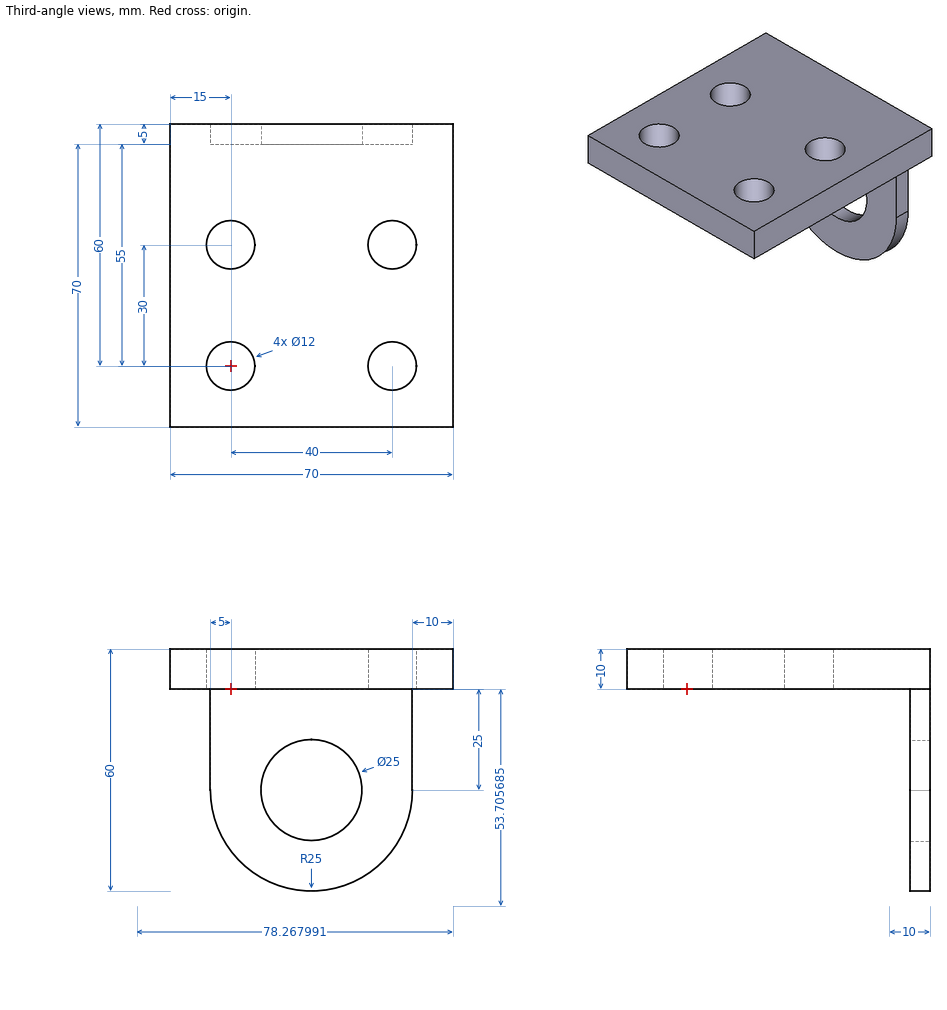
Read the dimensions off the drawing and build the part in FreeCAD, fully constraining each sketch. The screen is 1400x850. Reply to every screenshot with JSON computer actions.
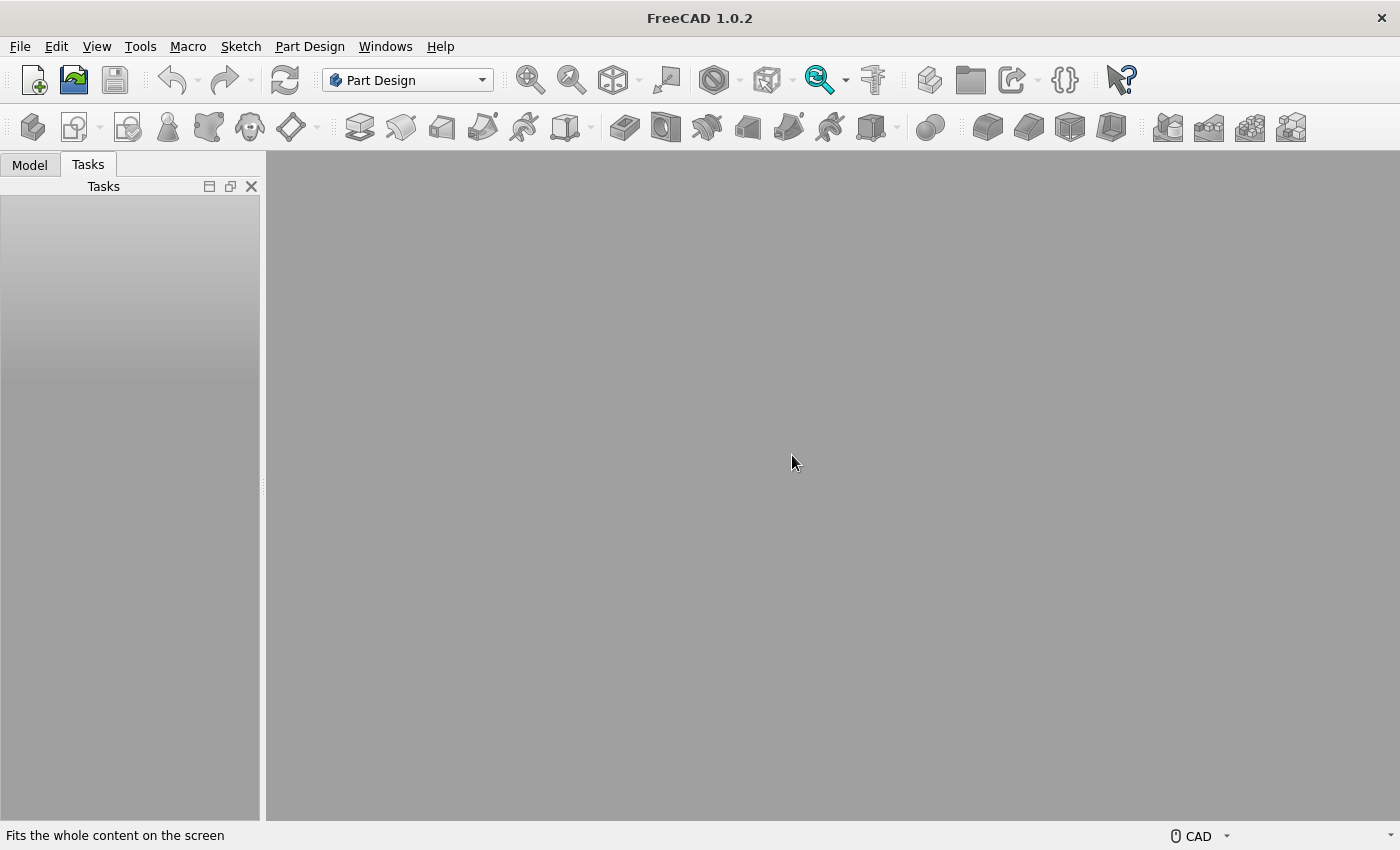
{"action": "key", "text": "ctrl+n"}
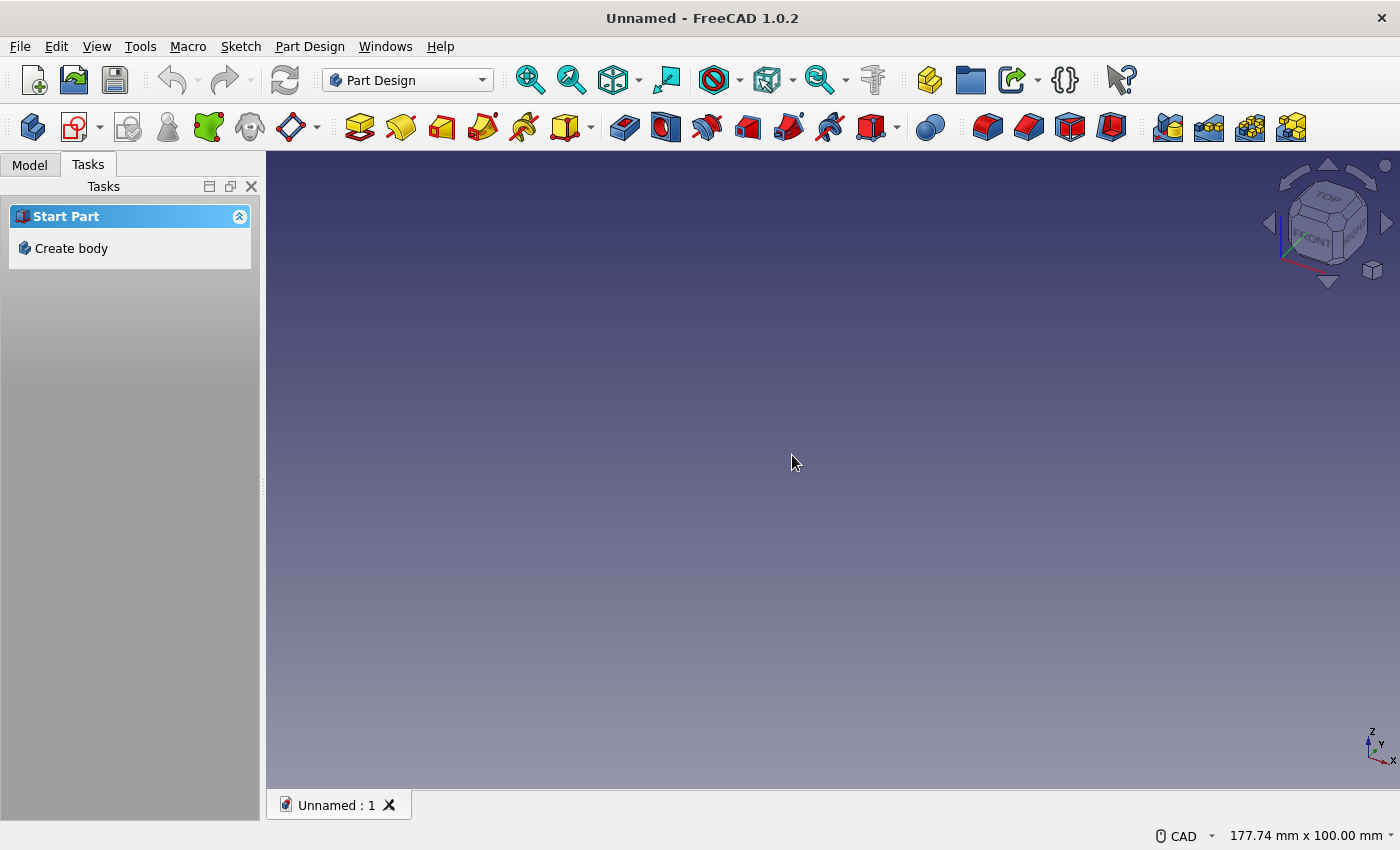
{"action": "left_click", "coordinate": [74, 128]}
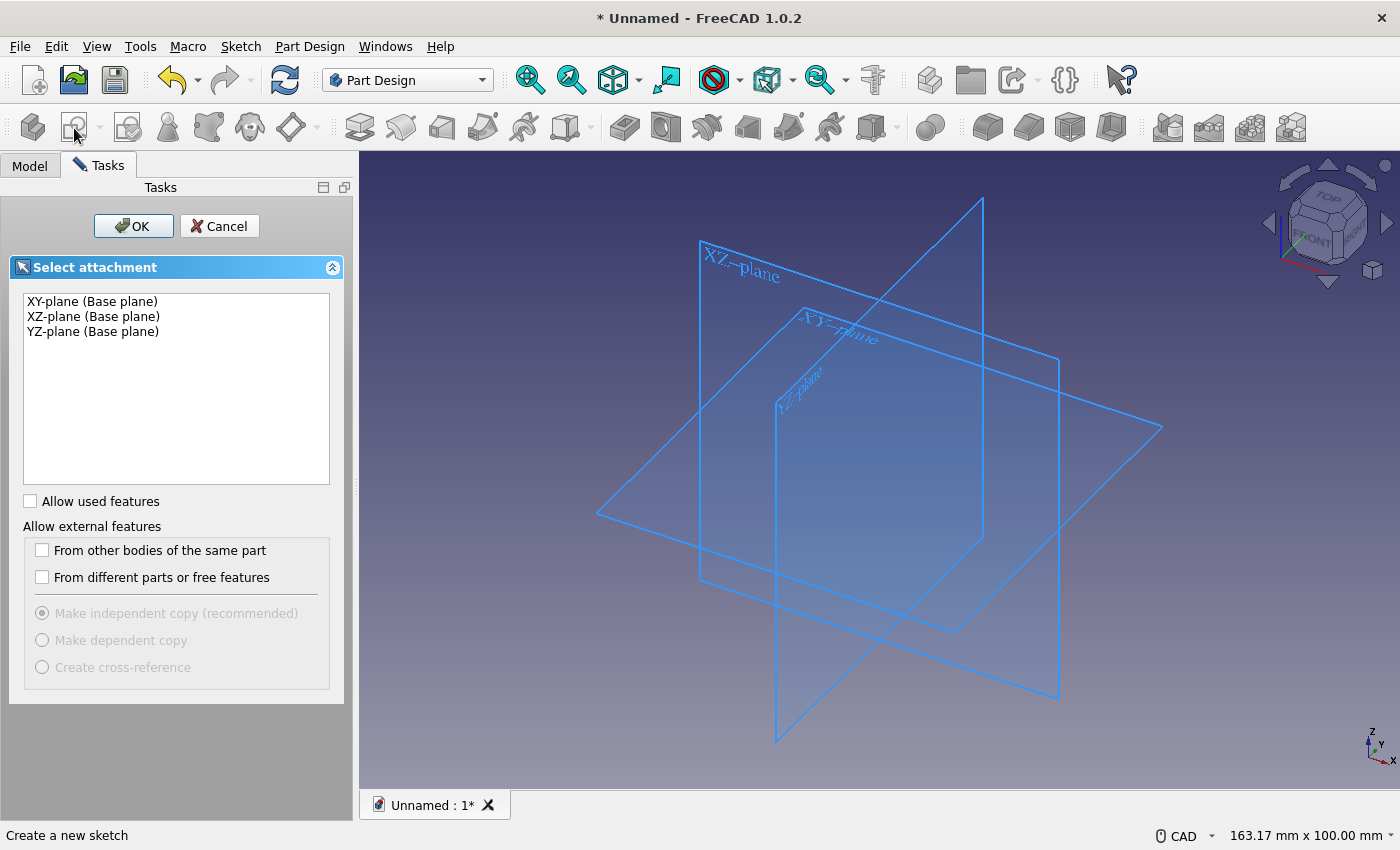
{"action": "left_click", "coordinate": [84, 302]}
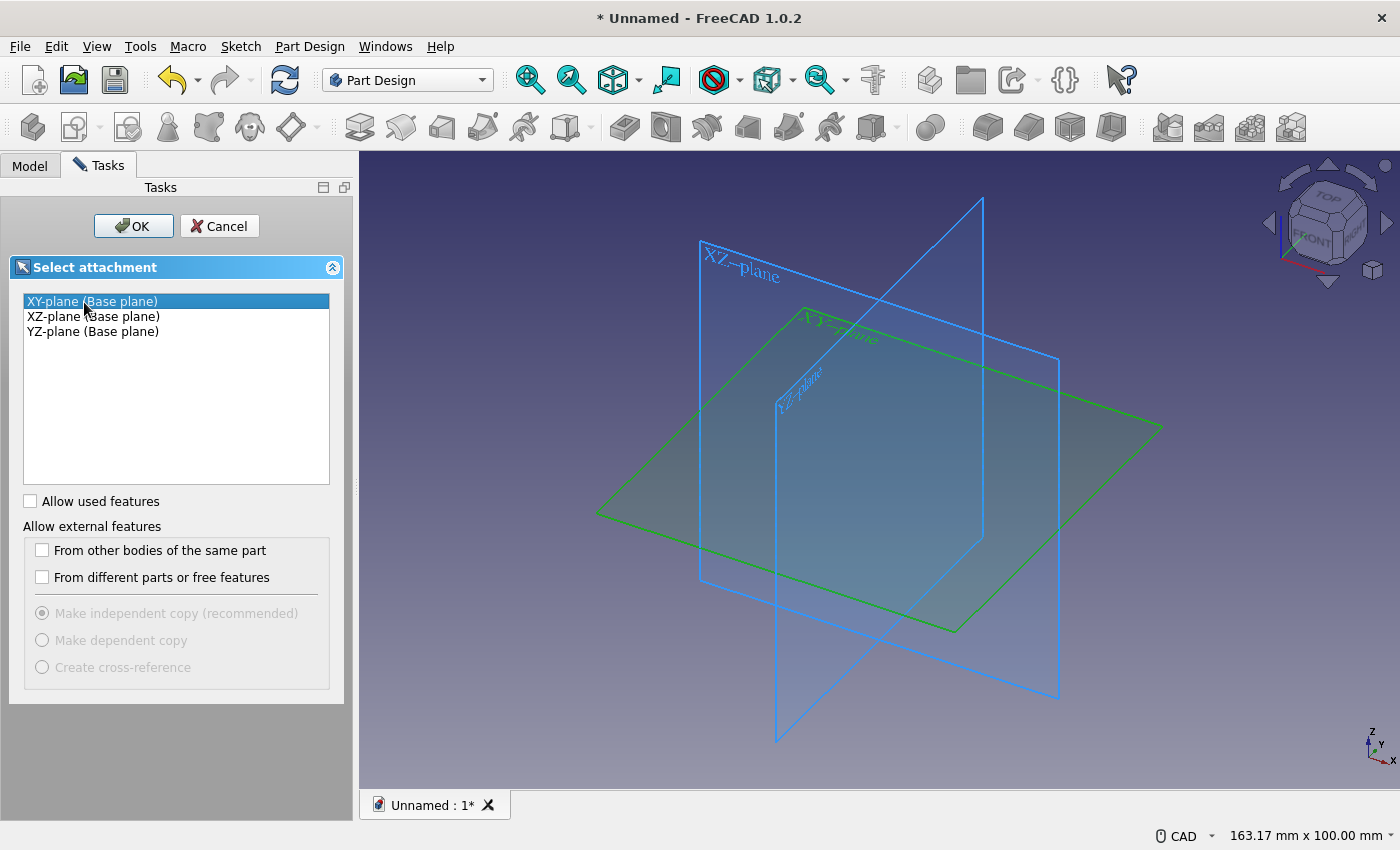
{"action": "left_click", "coordinate": [134, 226]}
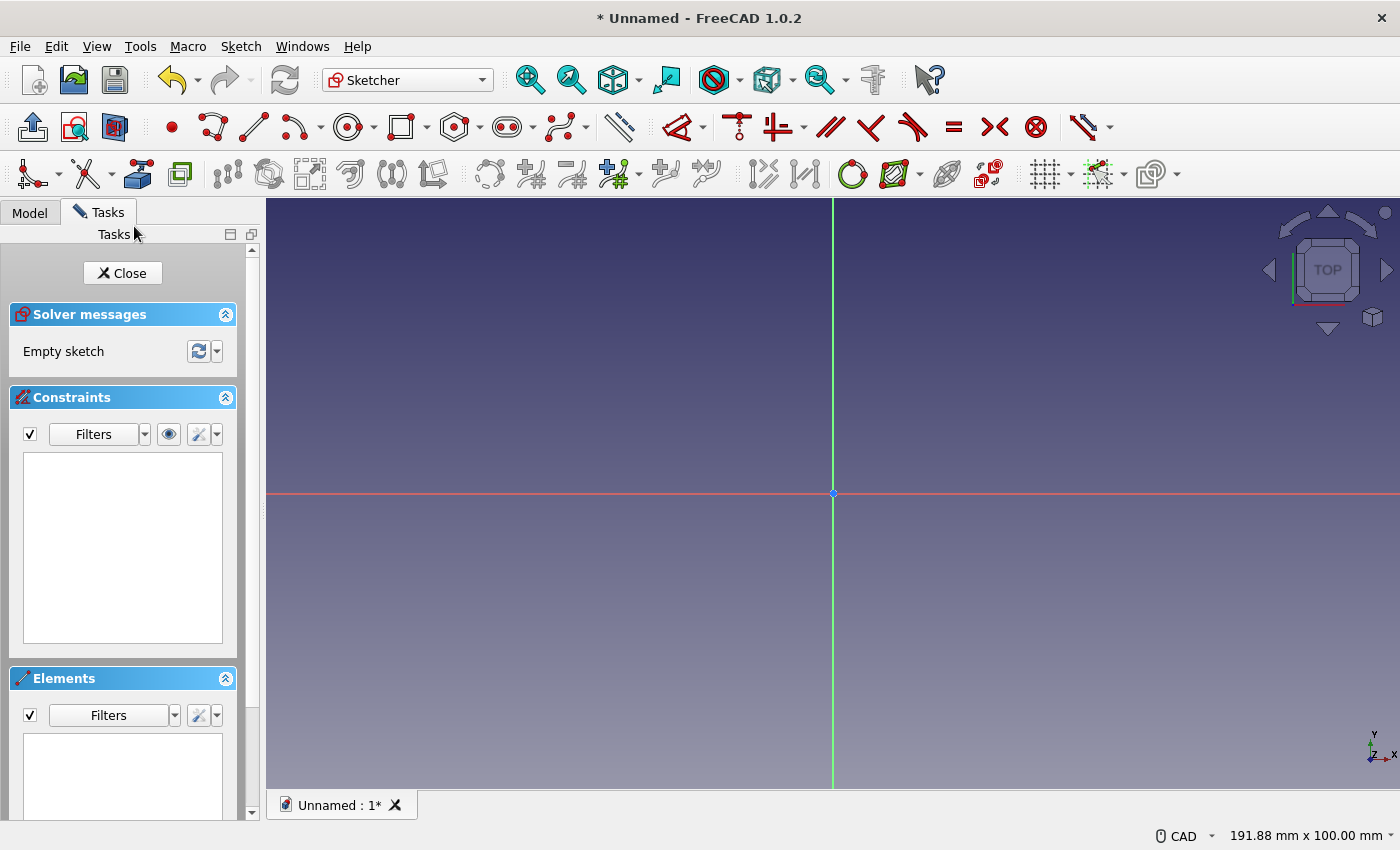
{"action": "scroll", "coordinate": [294, 761], "scroll_direction": "down", "scroll_amount": 1}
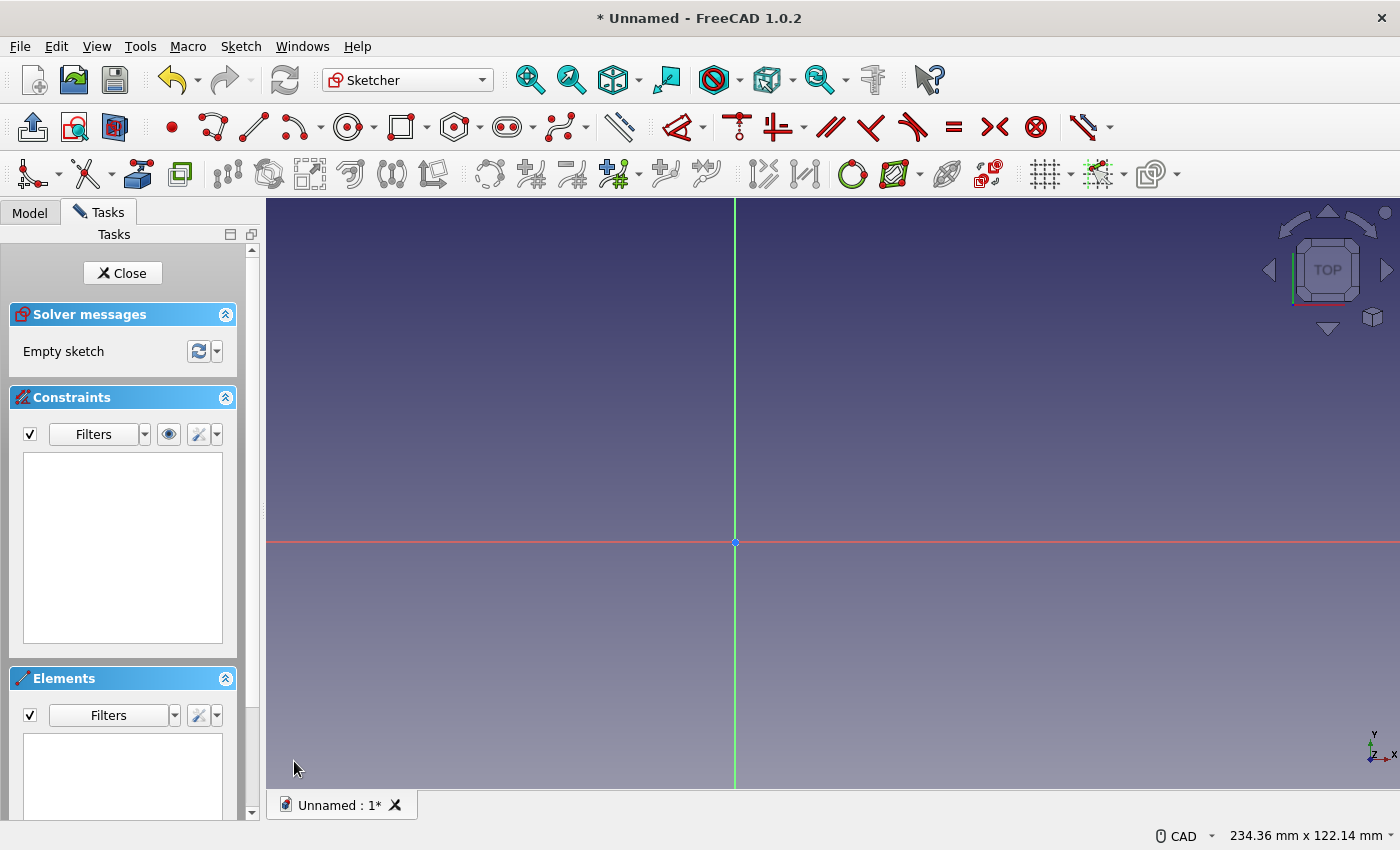
{"action": "left_click", "coordinate": [400, 128]}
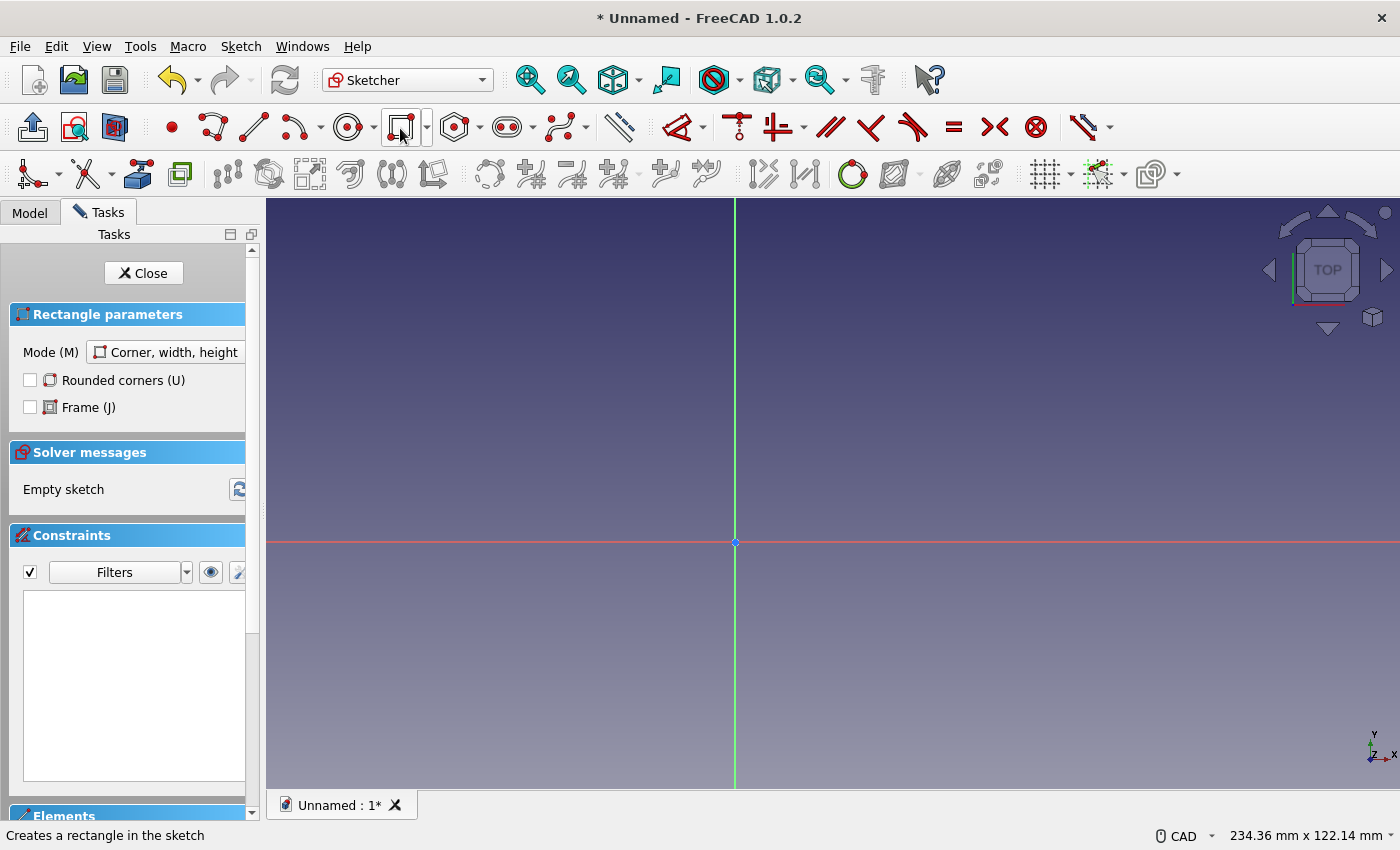
{"action": "left_click", "coordinate": [663, 276]}
{"action": "left_click", "coordinate": [1001, 615]}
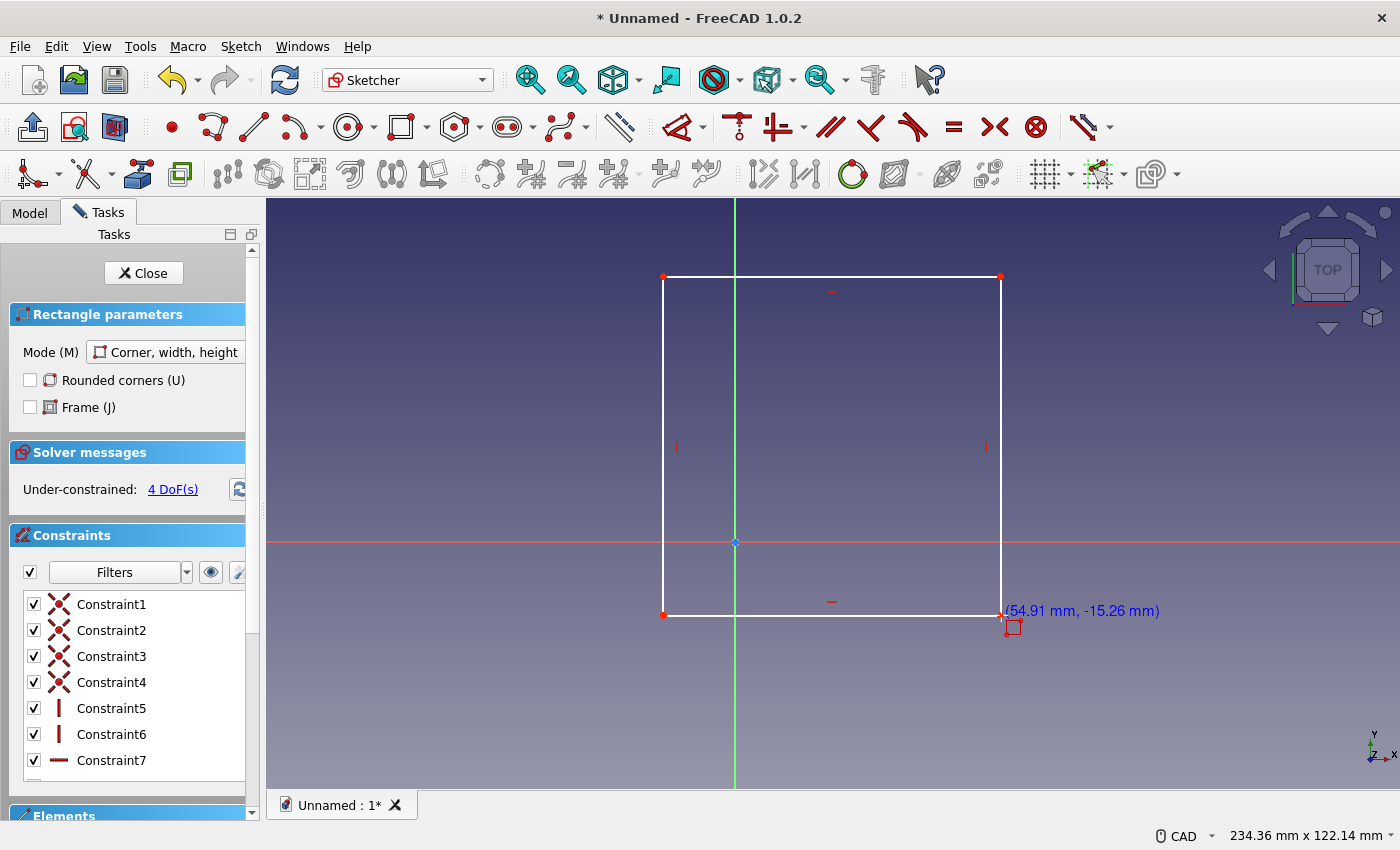
{"action": "left_click", "coordinate": [348, 128]}